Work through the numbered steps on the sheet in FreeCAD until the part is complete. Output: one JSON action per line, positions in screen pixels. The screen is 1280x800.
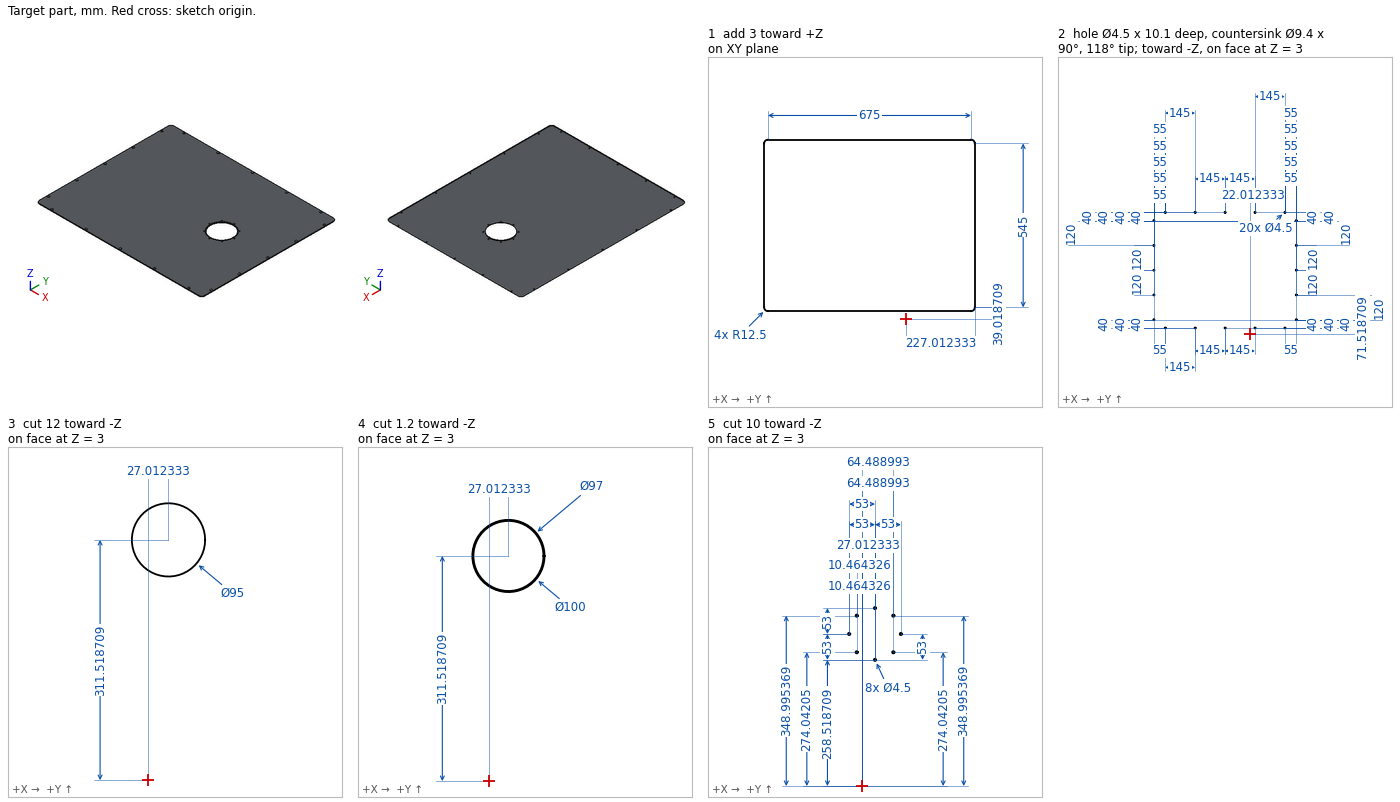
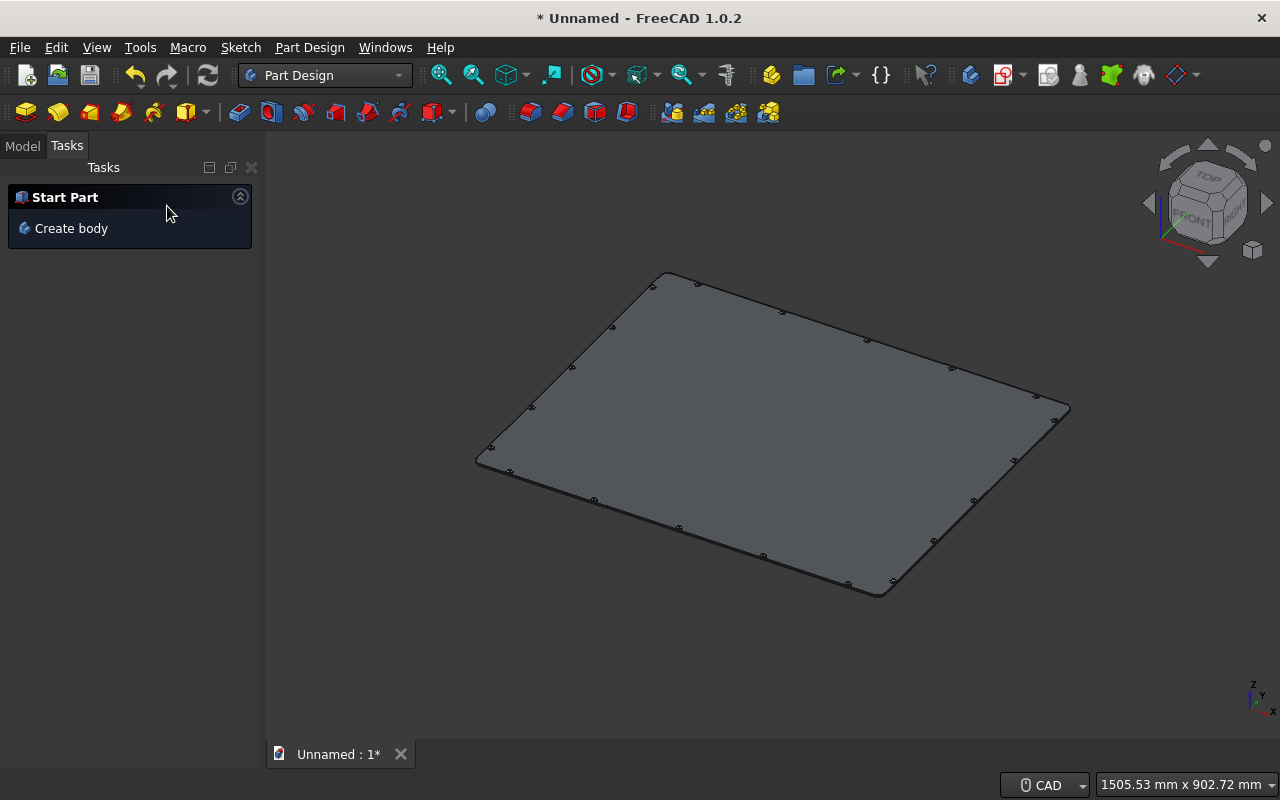
{"action": "left_click", "coordinate": [773, 433]}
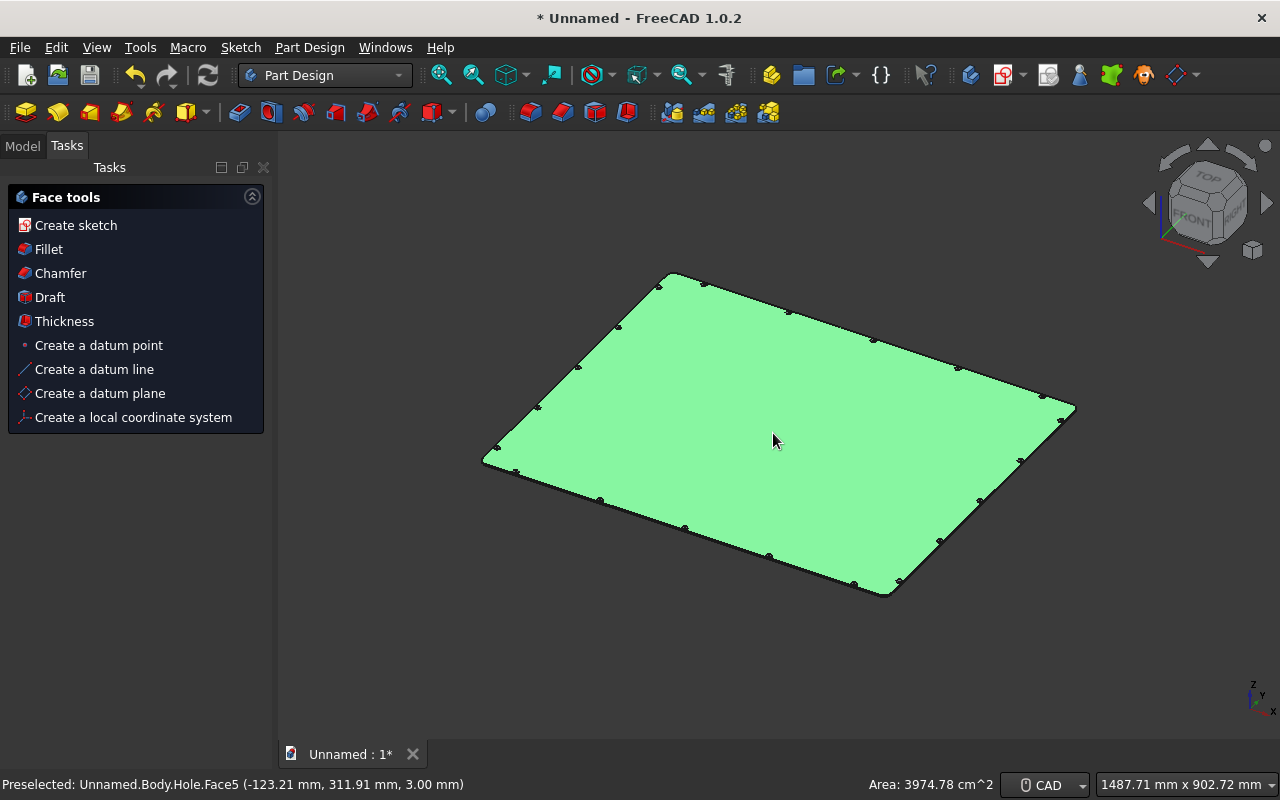
{"action": "left_click", "coordinate": [1004, 76]}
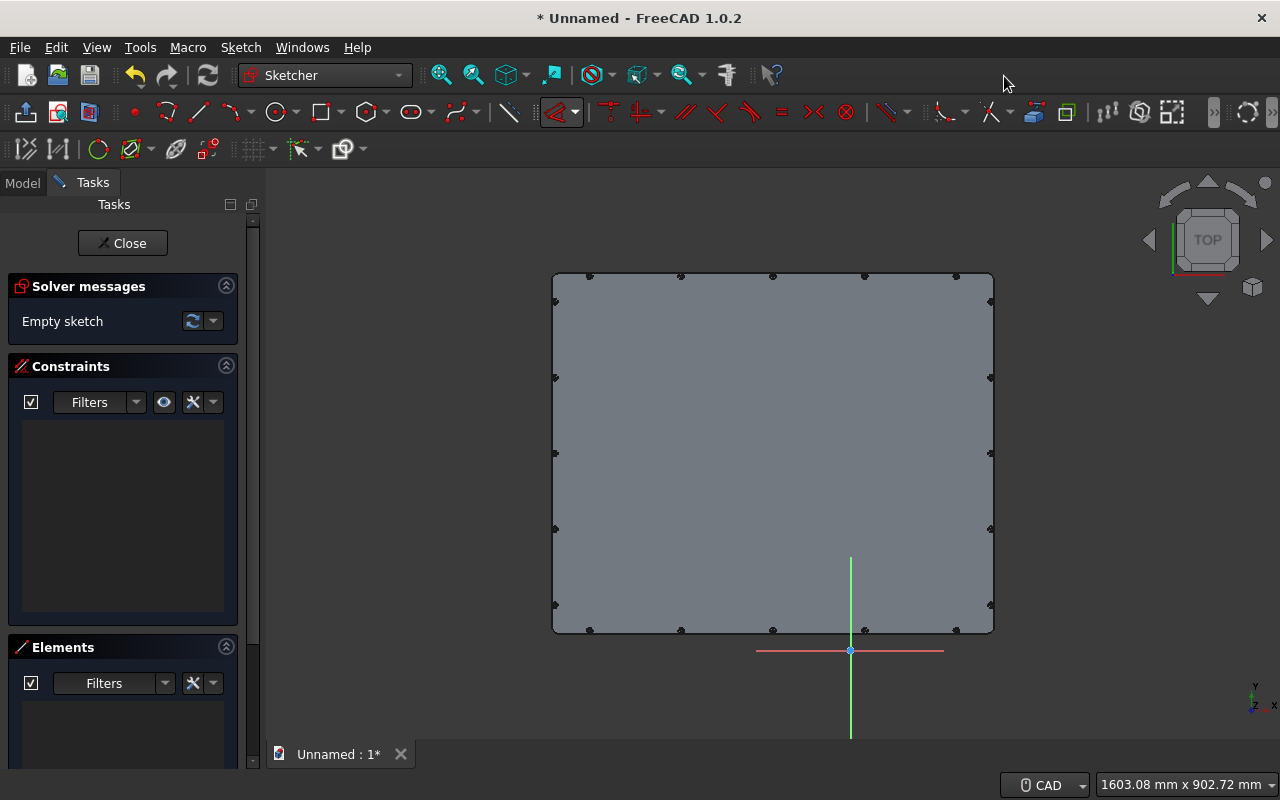
{"action": "scroll", "coordinate": [900, 454], "scroll_direction": "up", "scroll_amount": 9}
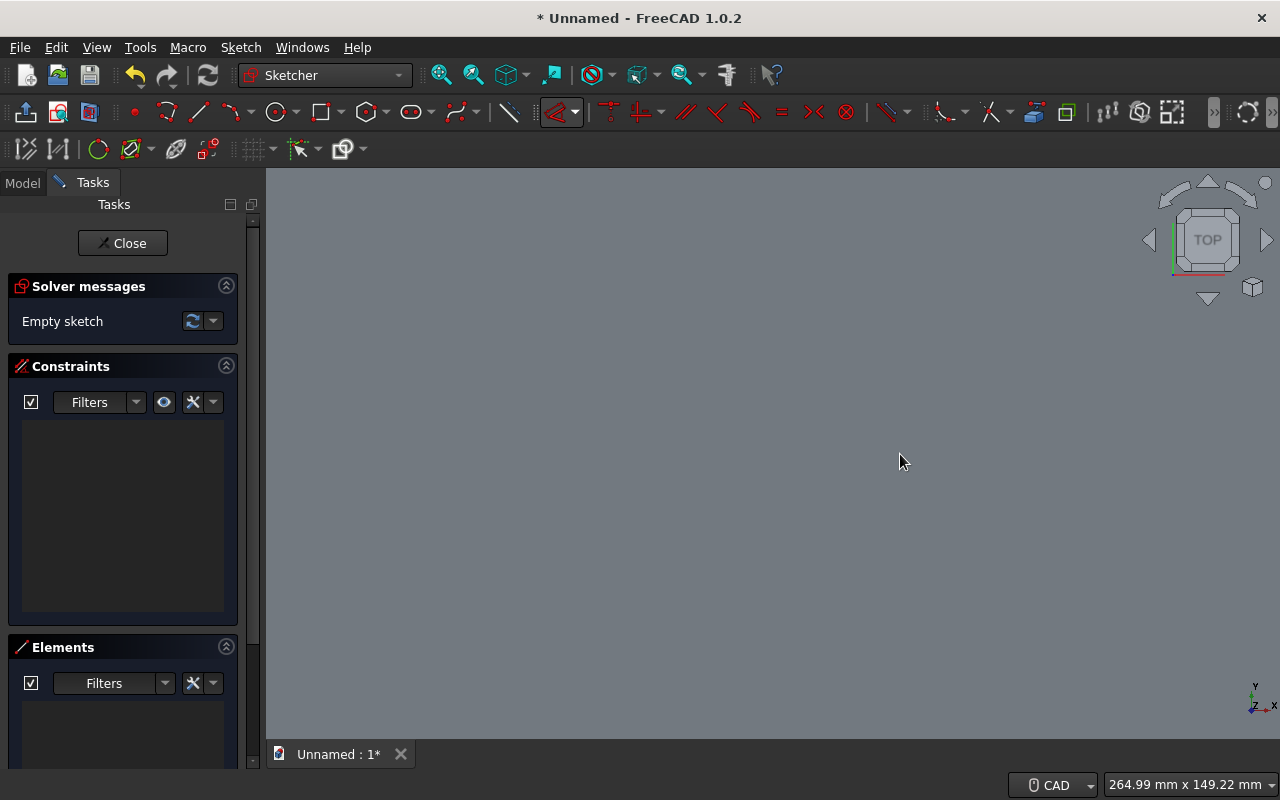
{"action": "left_click", "coordinate": [276, 112]}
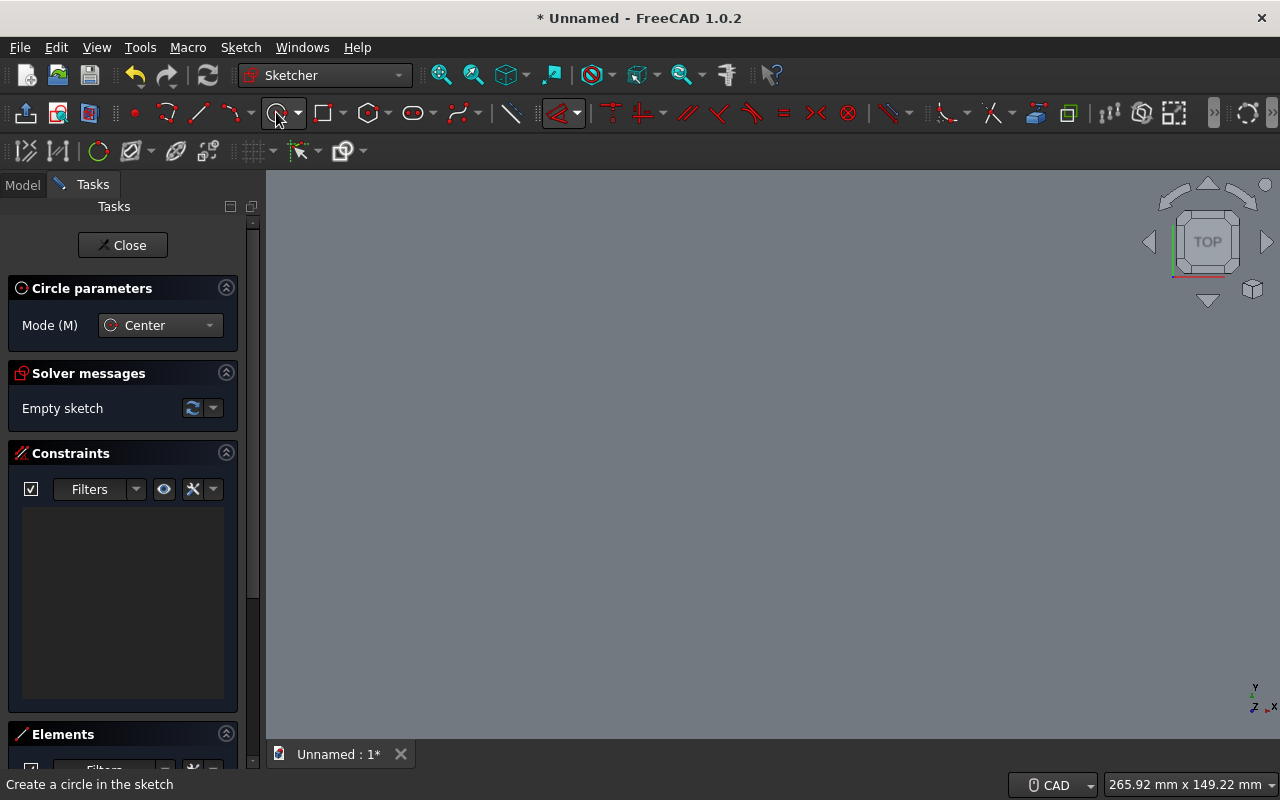
{"action": "left_click", "coordinate": [703, 449]}
{"action": "left_click", "coordinate": [831, 321]}
{"action": "key", "text": "Escape"}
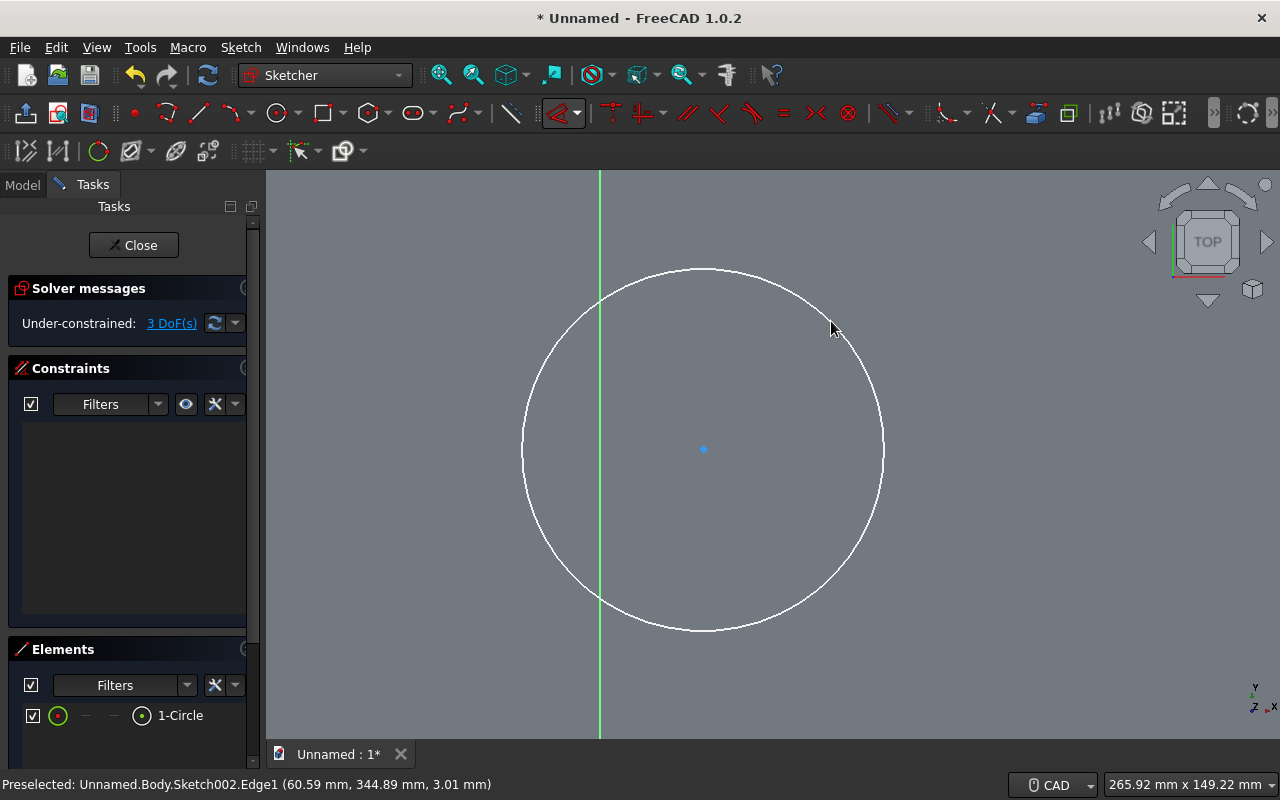
{"action": "left_click", "coordinate": [831, 322]}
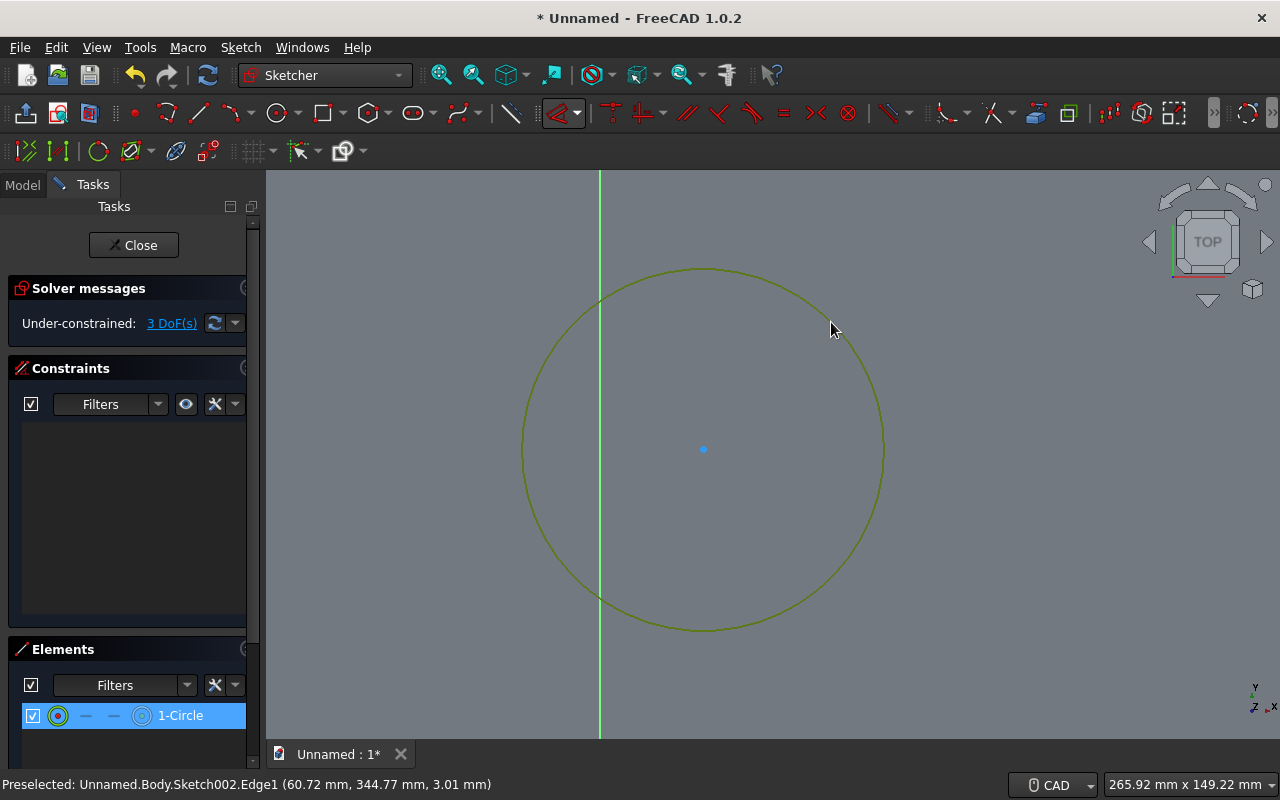
{"action": "key", "text": "k o"}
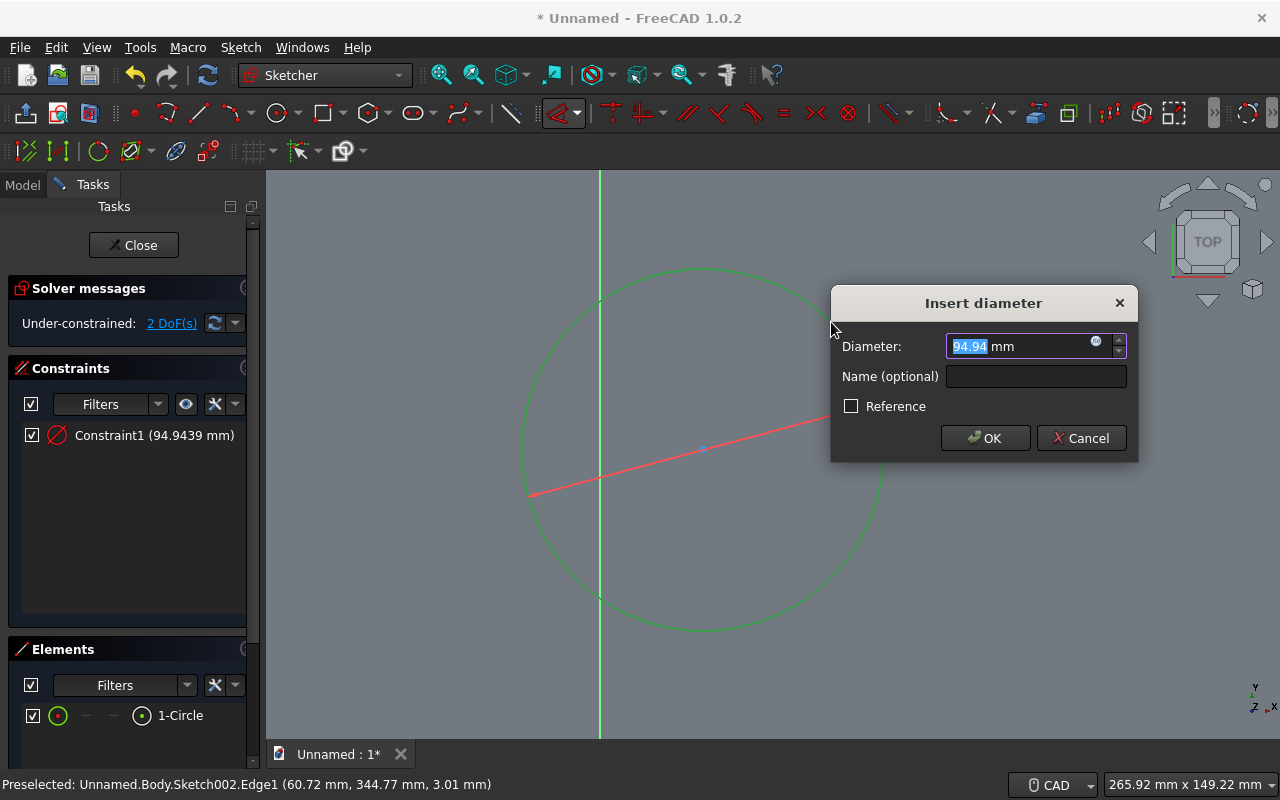
{"action": "type", "text": "95"}
{"action": "key", "text": "Return"}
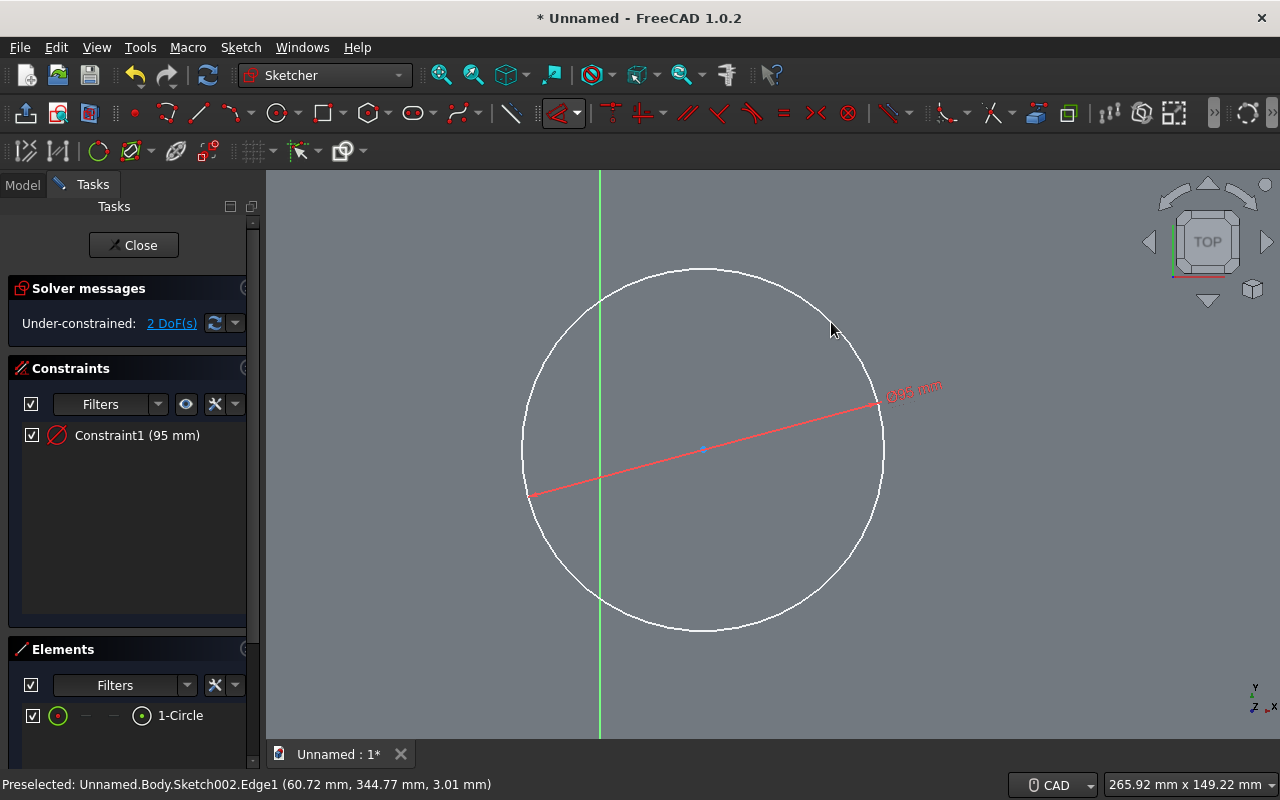
{"action": "left_click", "coordinate": [703, 450]}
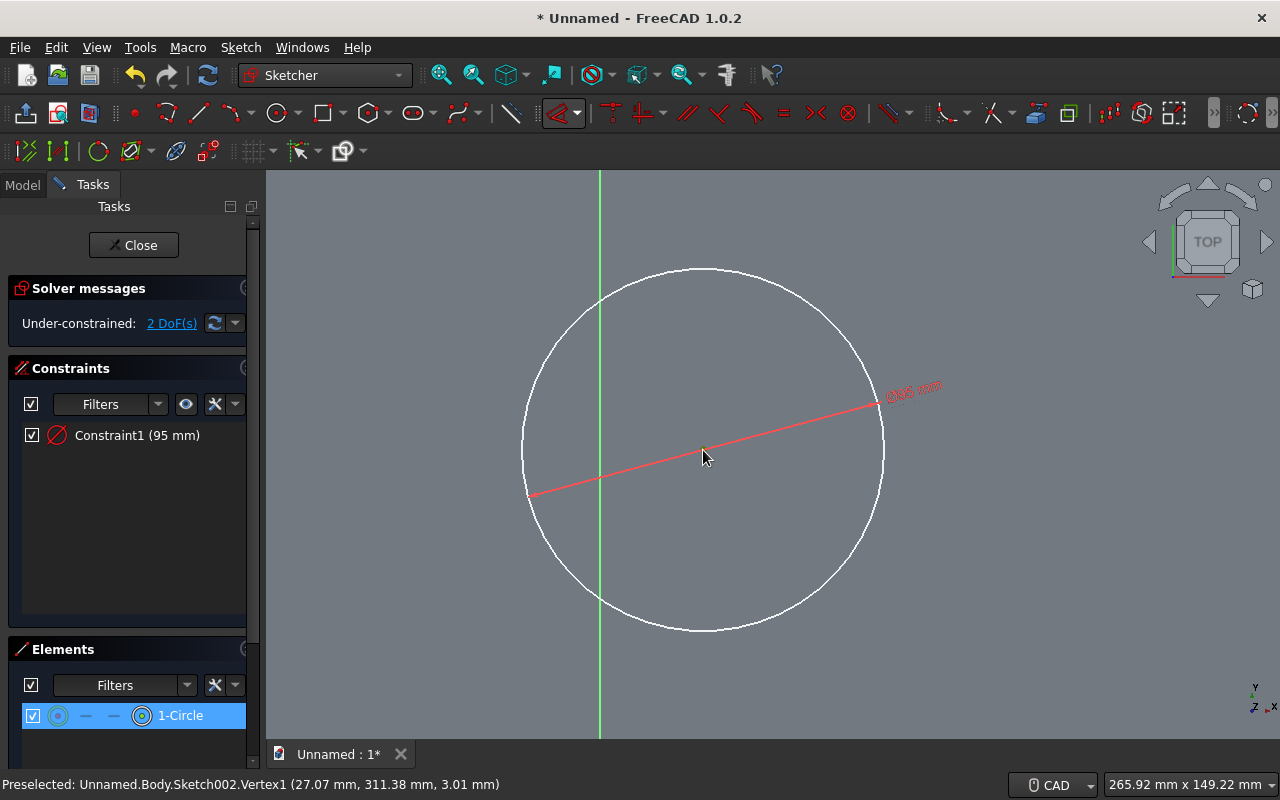
{"action": "key", "text": "l"}